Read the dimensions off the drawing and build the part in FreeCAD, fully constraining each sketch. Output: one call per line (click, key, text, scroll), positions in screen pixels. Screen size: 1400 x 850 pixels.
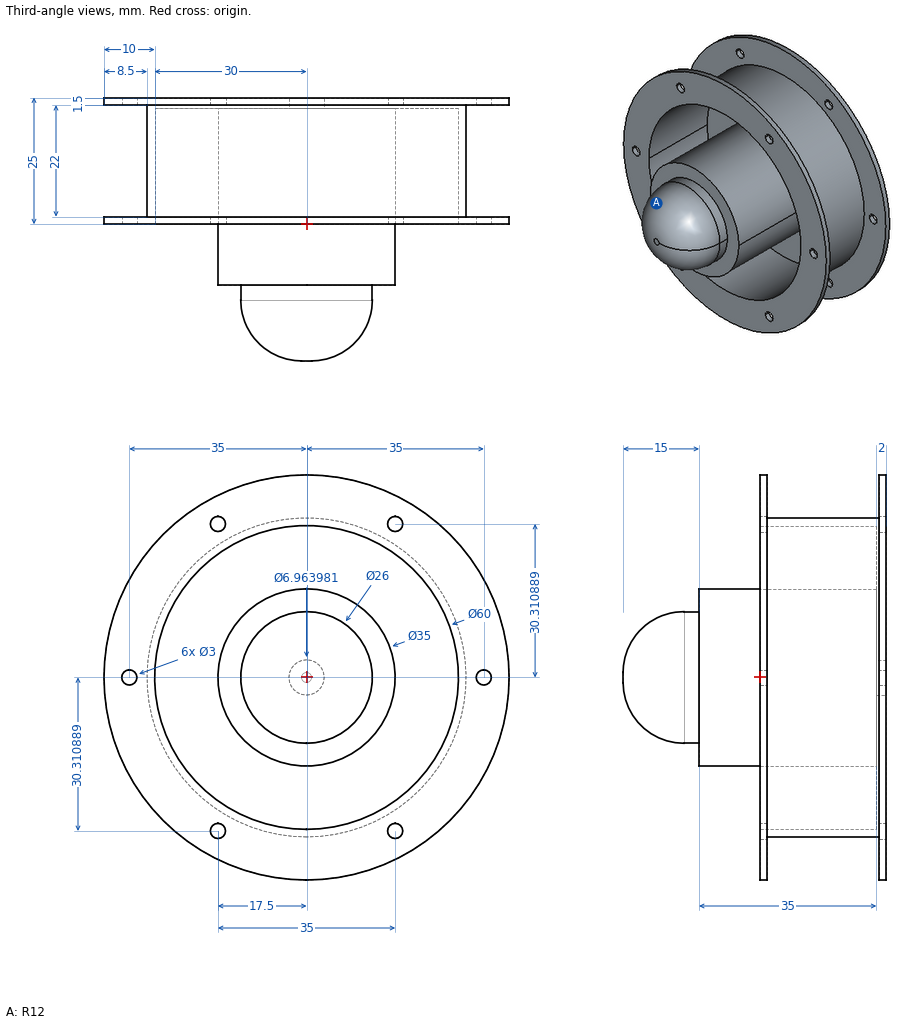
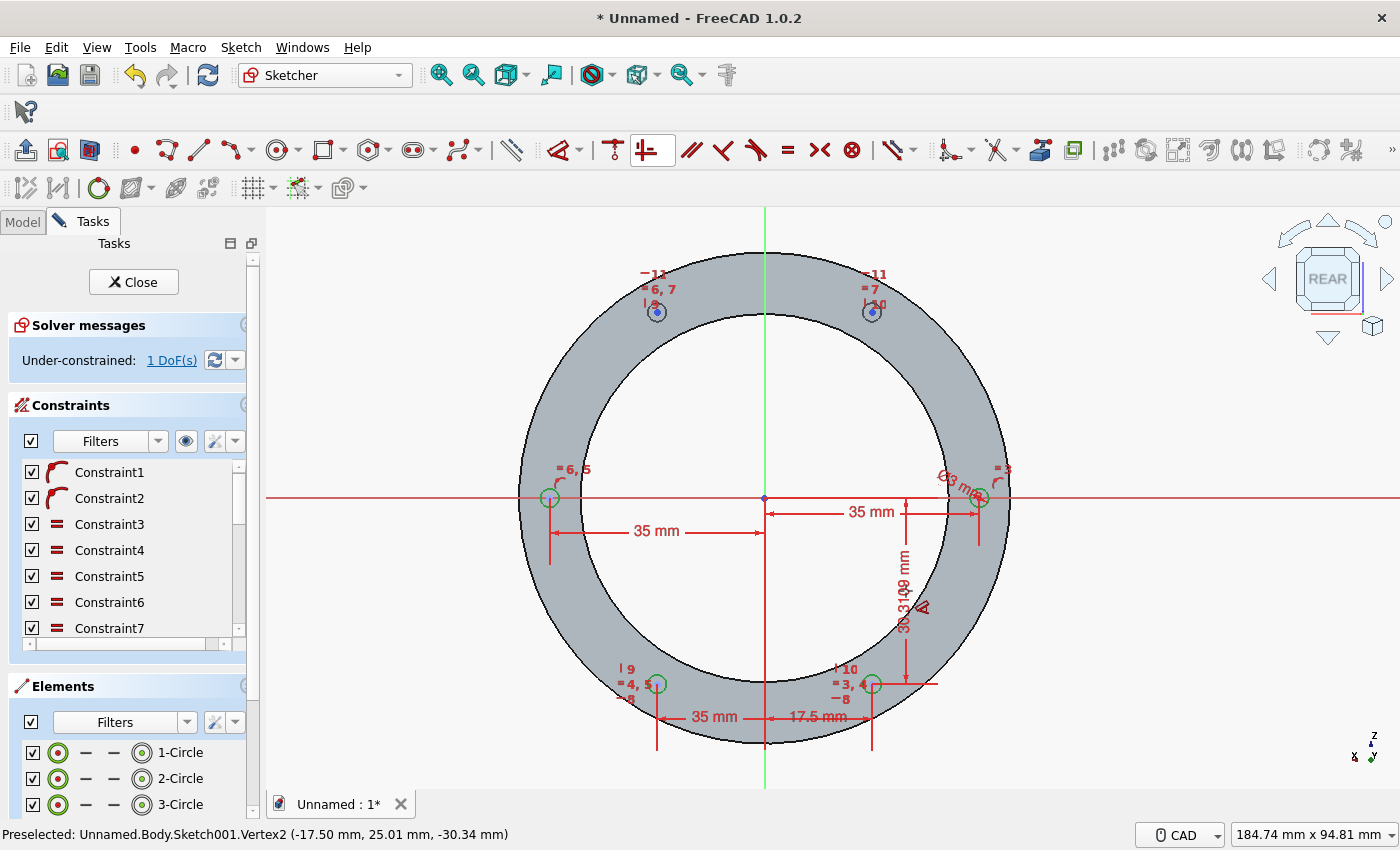
click(657, 312)
click(623, 405)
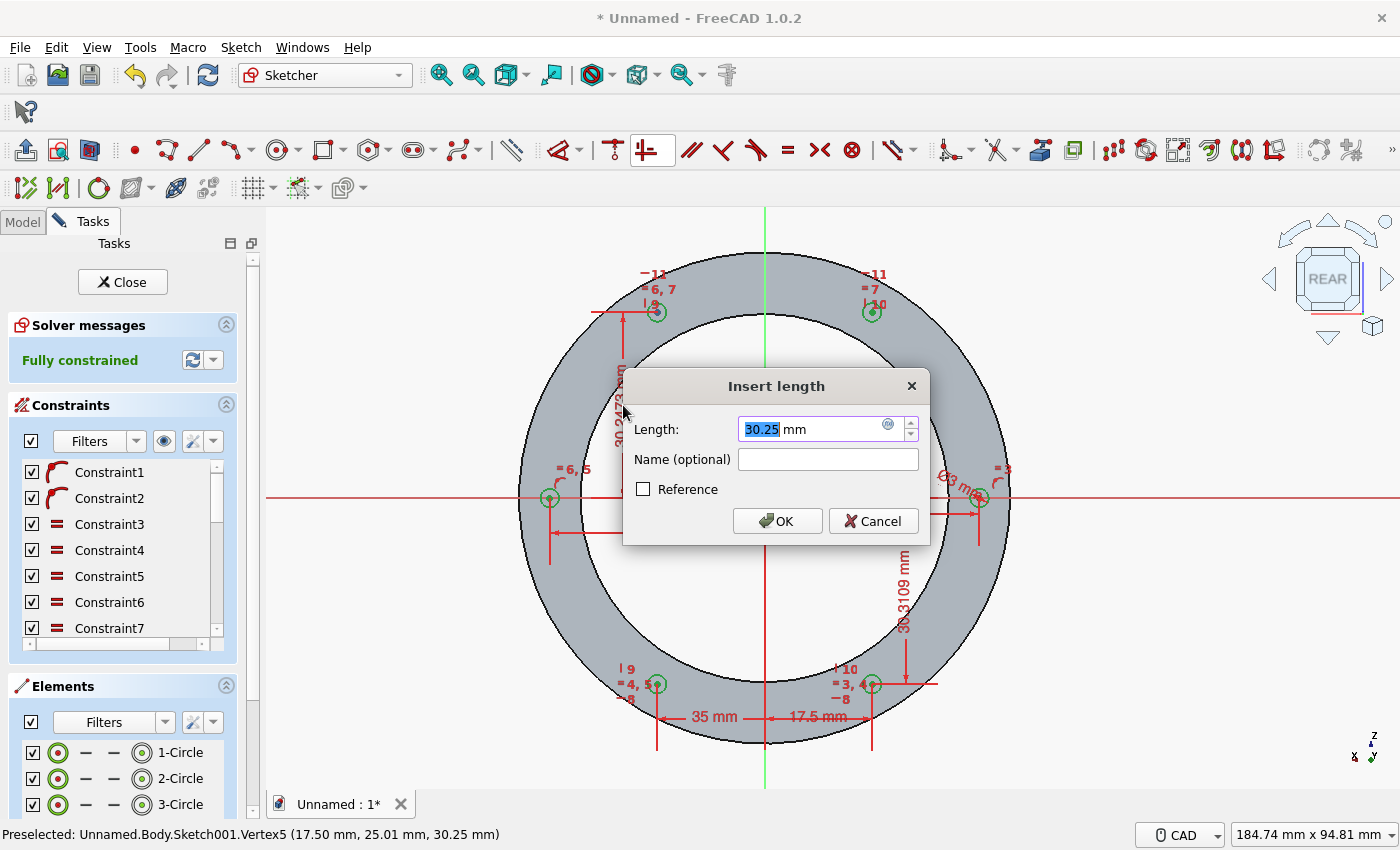
text(30.310889)
key(Return)
key(Escape)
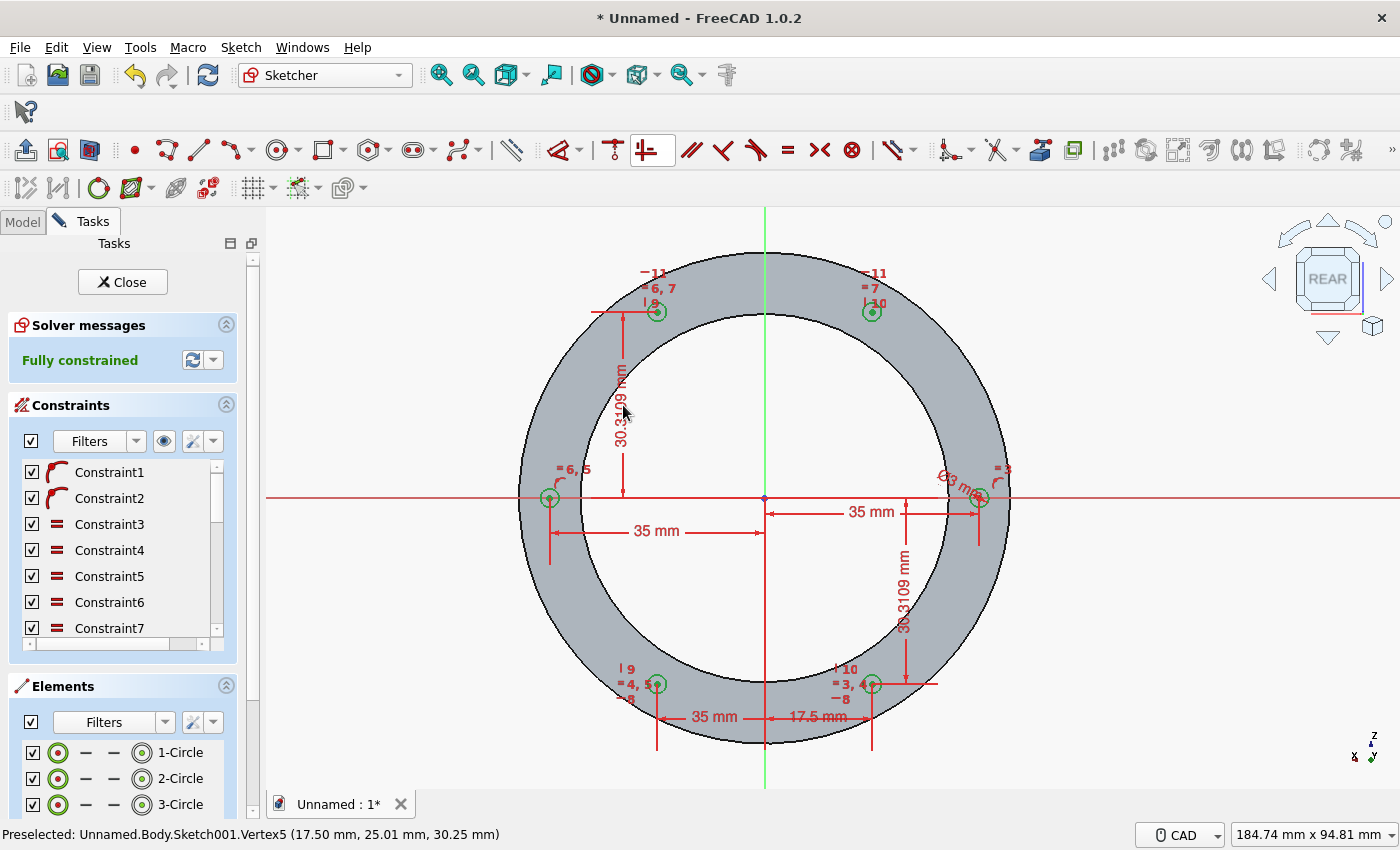
click(123, 282)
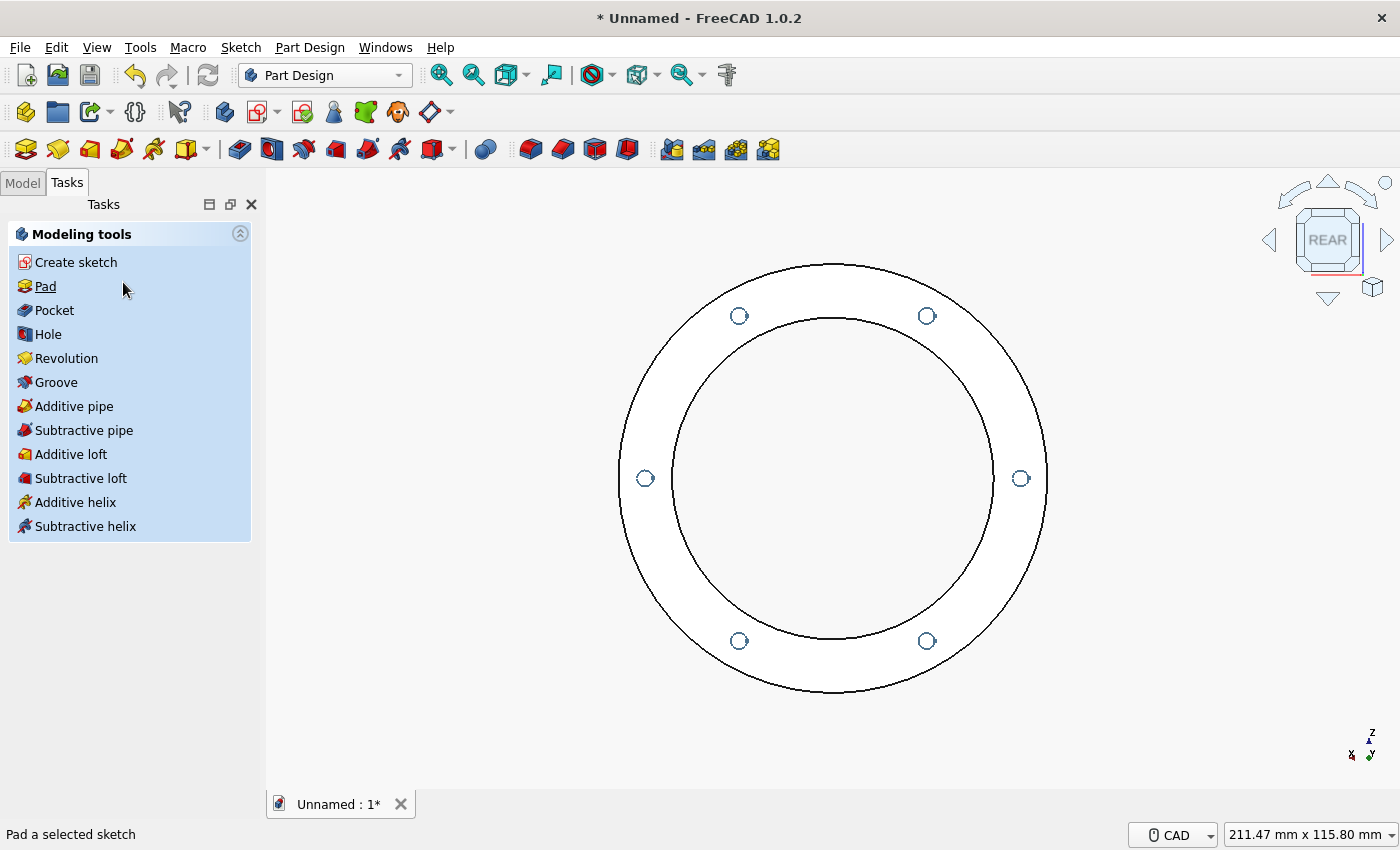
click(240, 150)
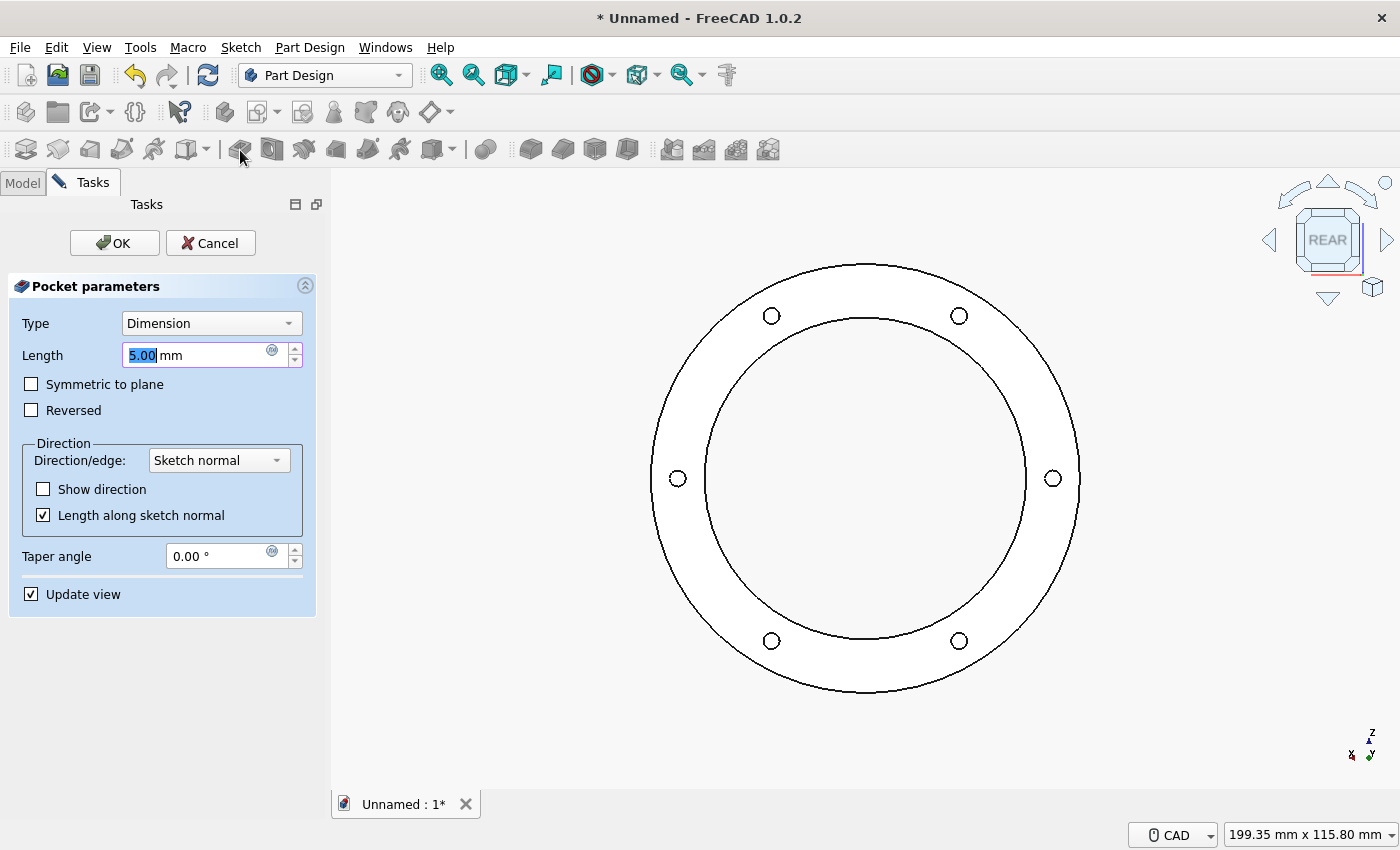
click(212, 324)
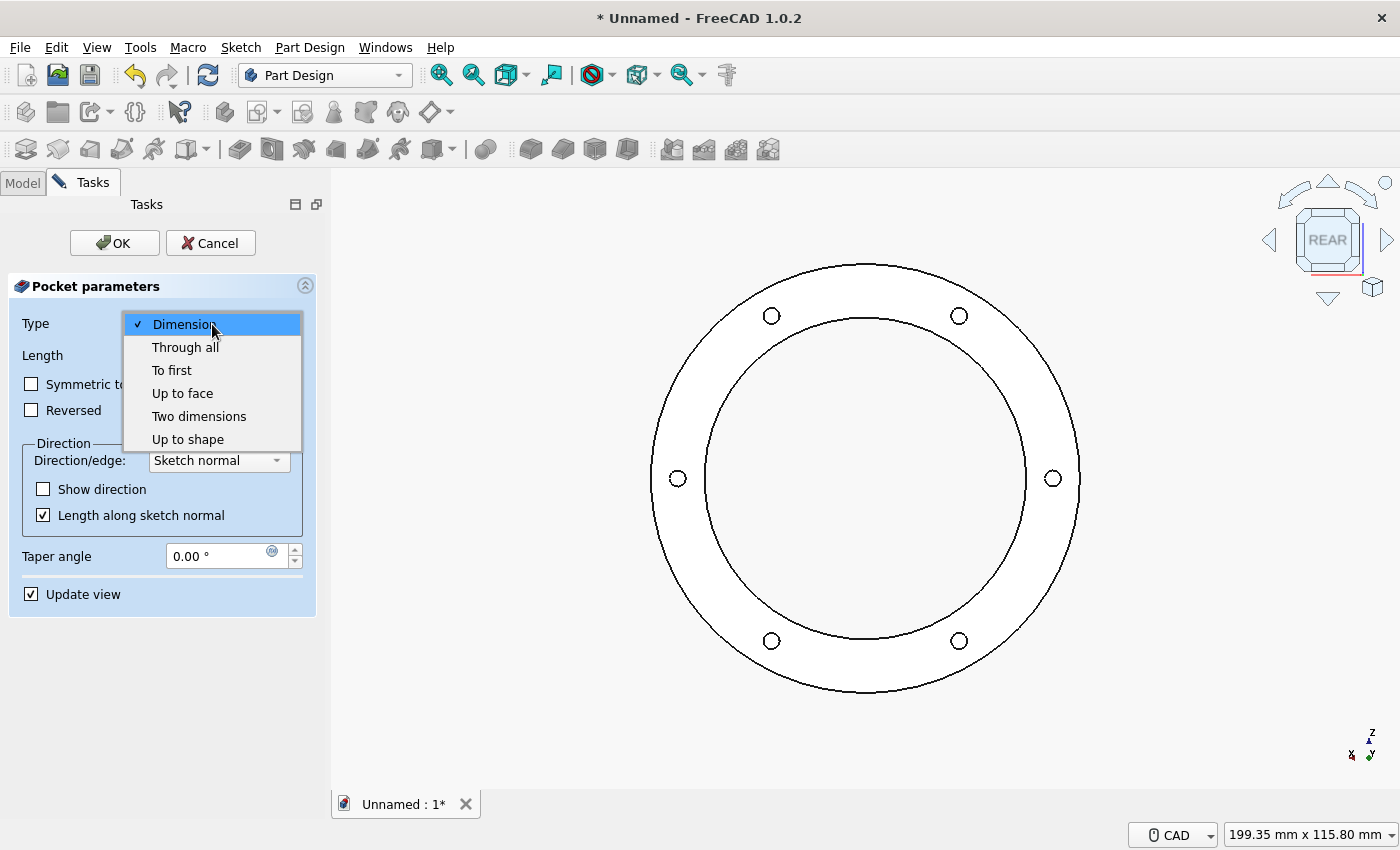
click(212, 348)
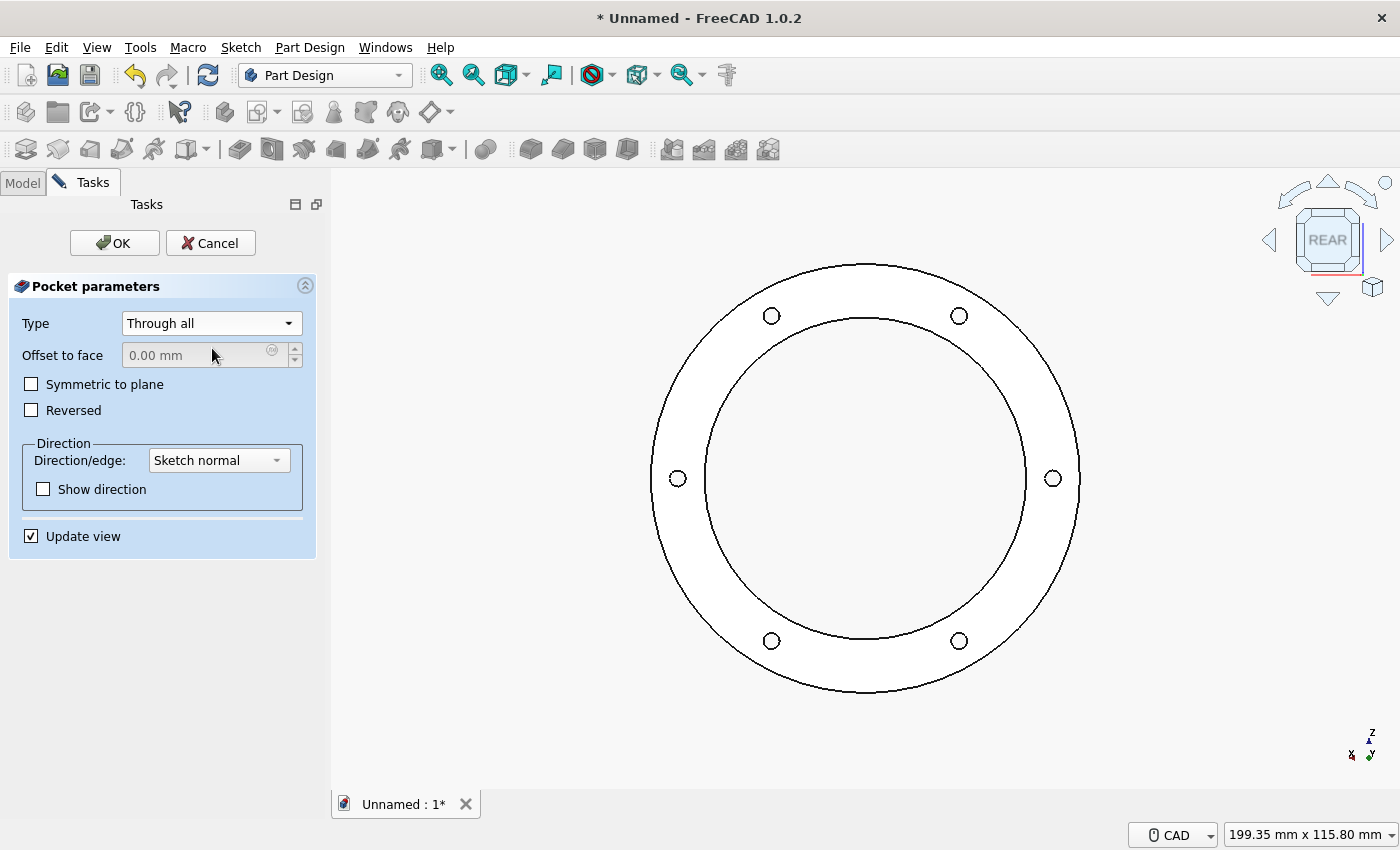
click(115, 243)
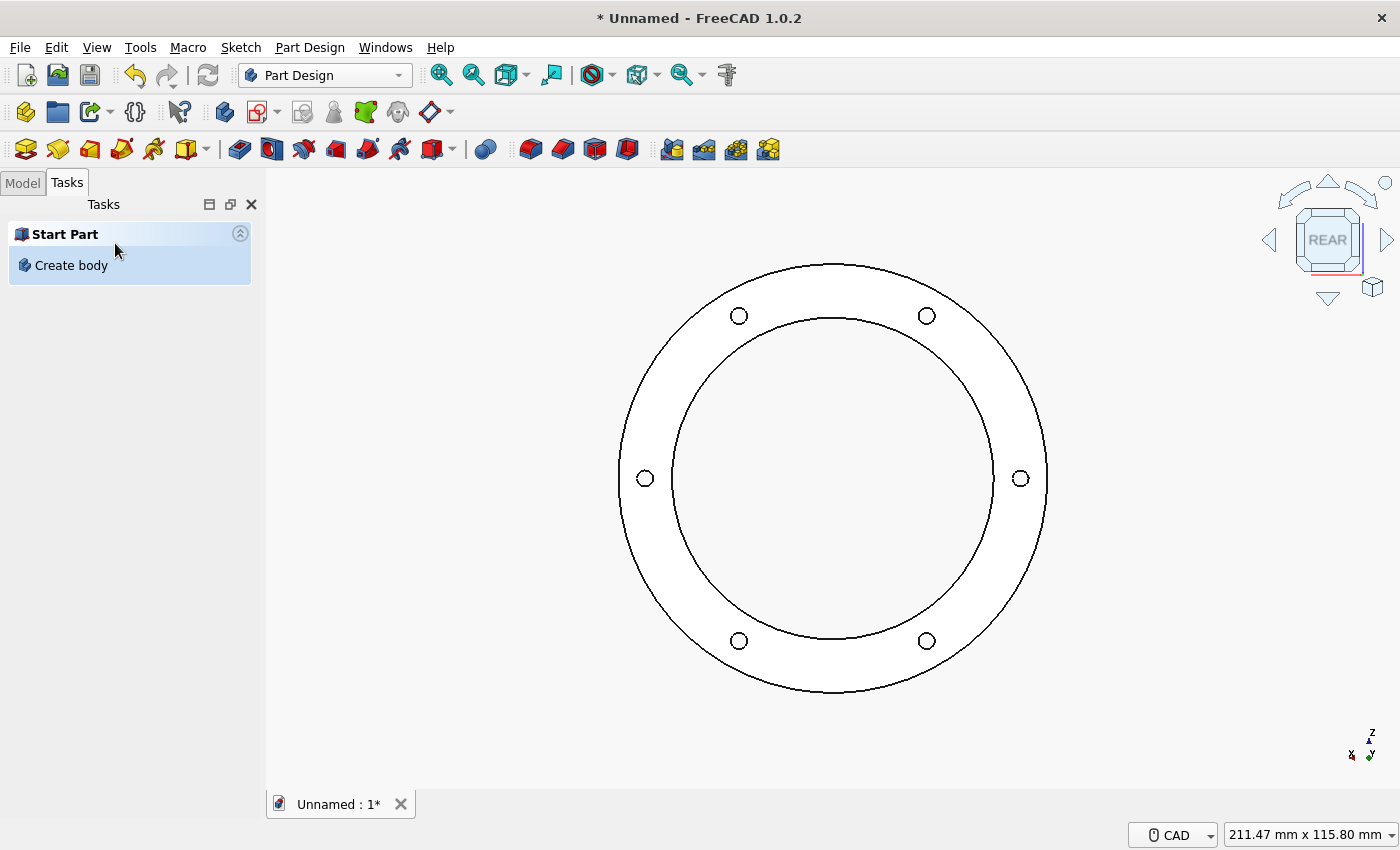
click(833, 294)